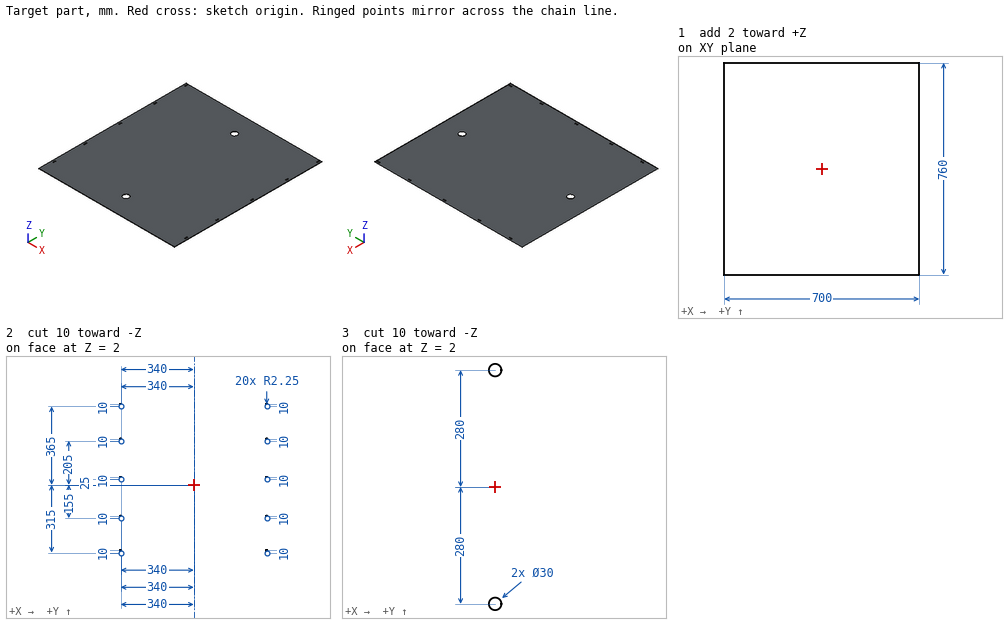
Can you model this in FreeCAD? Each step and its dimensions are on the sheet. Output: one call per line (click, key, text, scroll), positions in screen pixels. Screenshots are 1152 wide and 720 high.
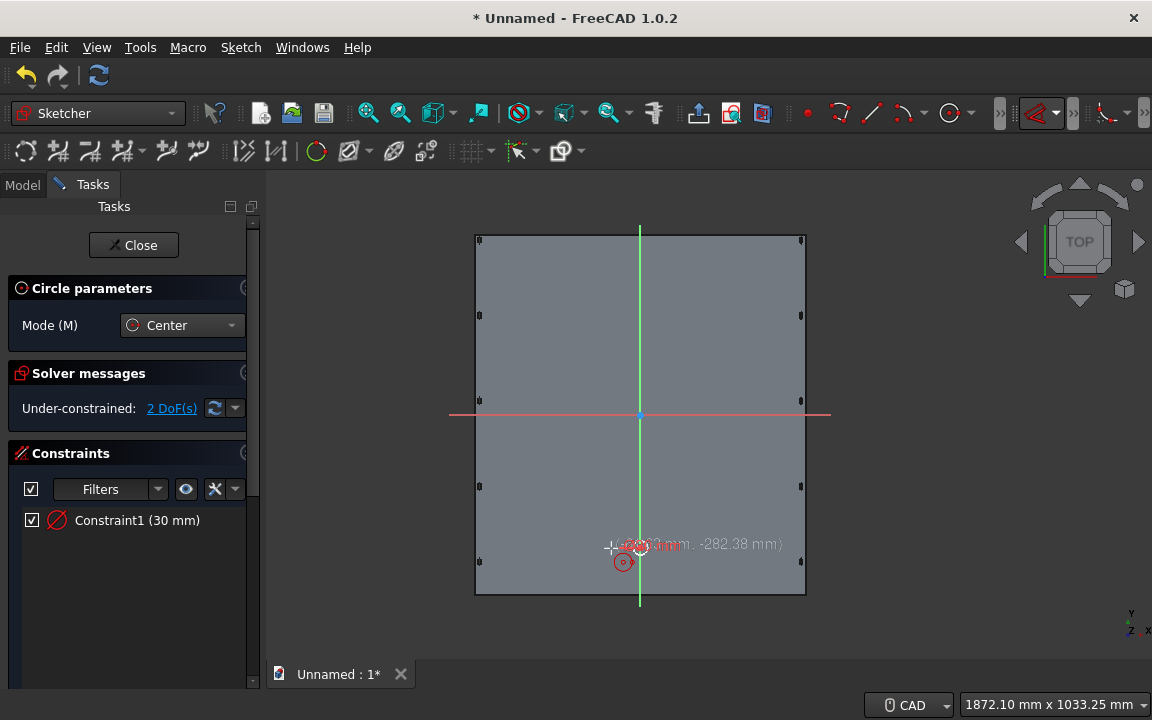
scroll(640, 283, up, 6)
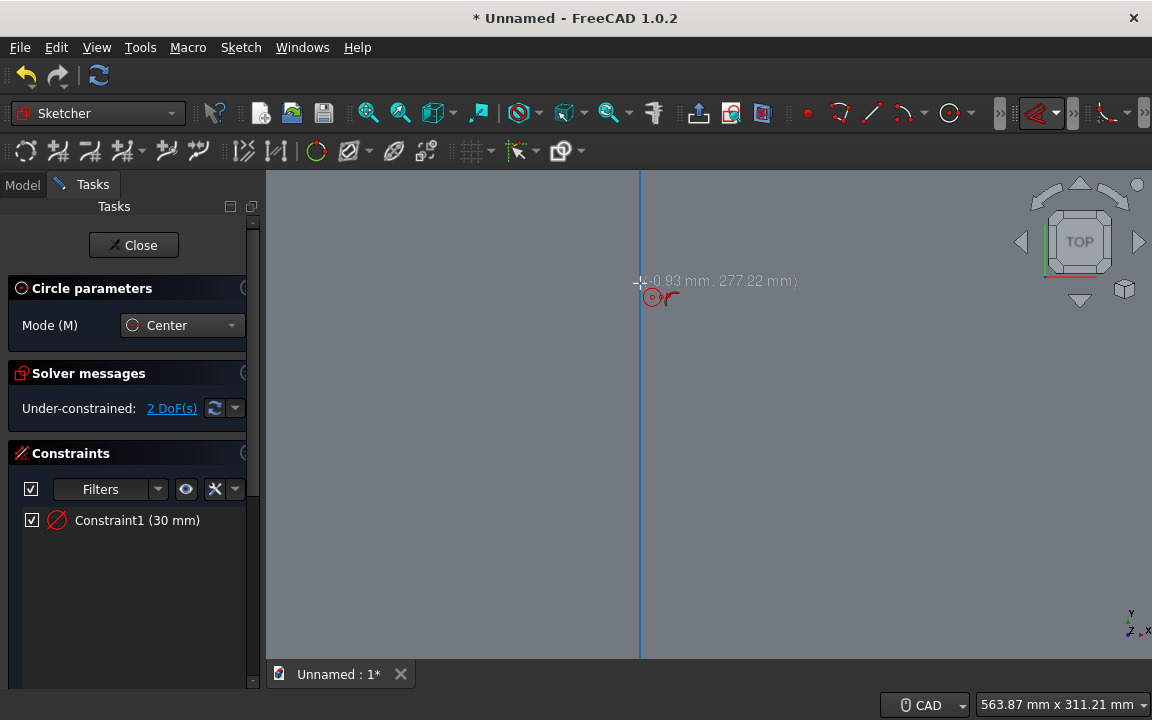
click(640, 281)
move(657, 265)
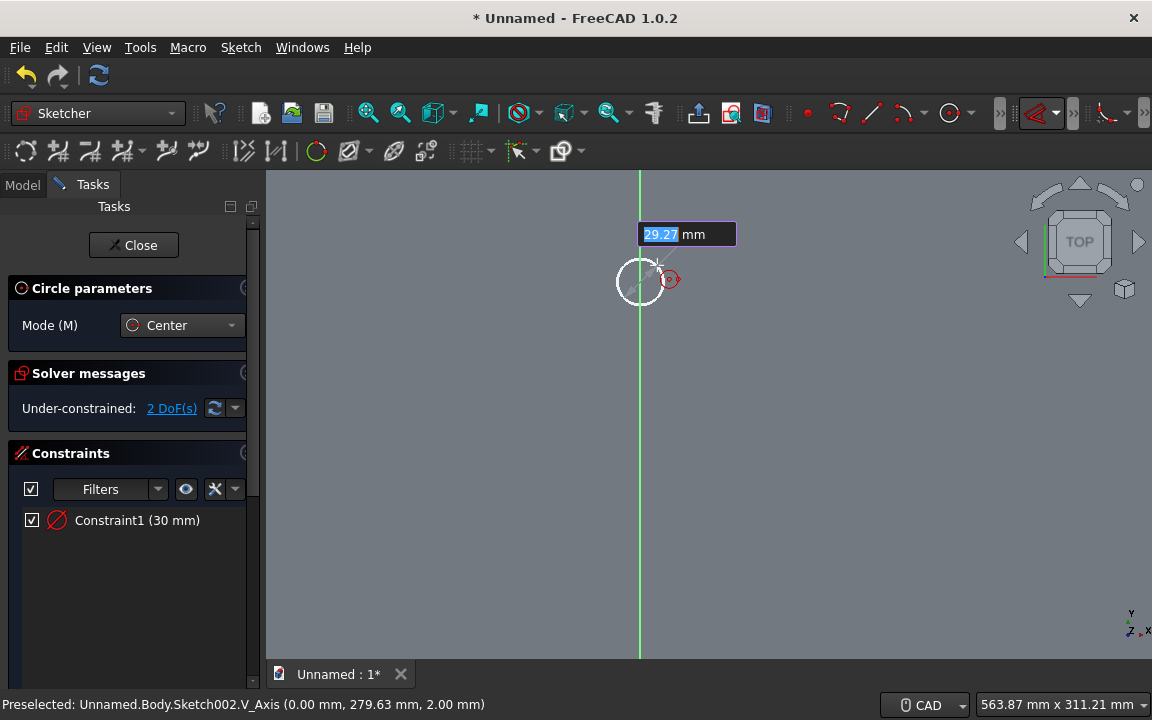
text(30)
key(Return)
key(Escape)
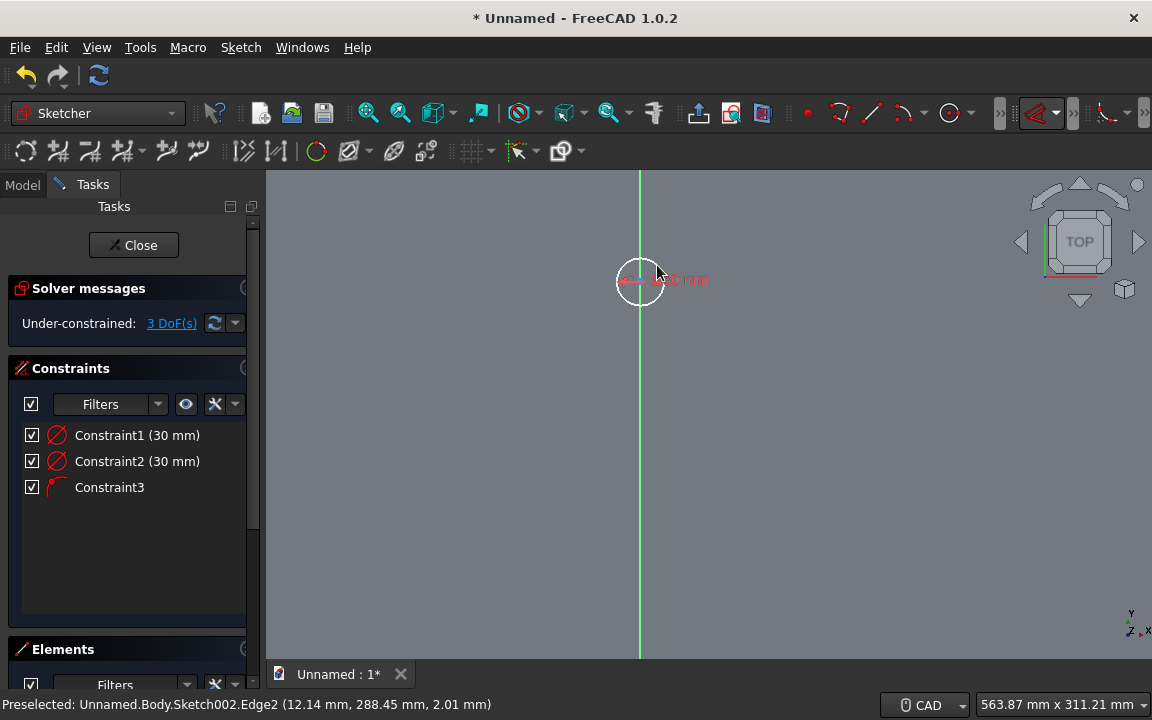
scroll(641, 282, down, 6)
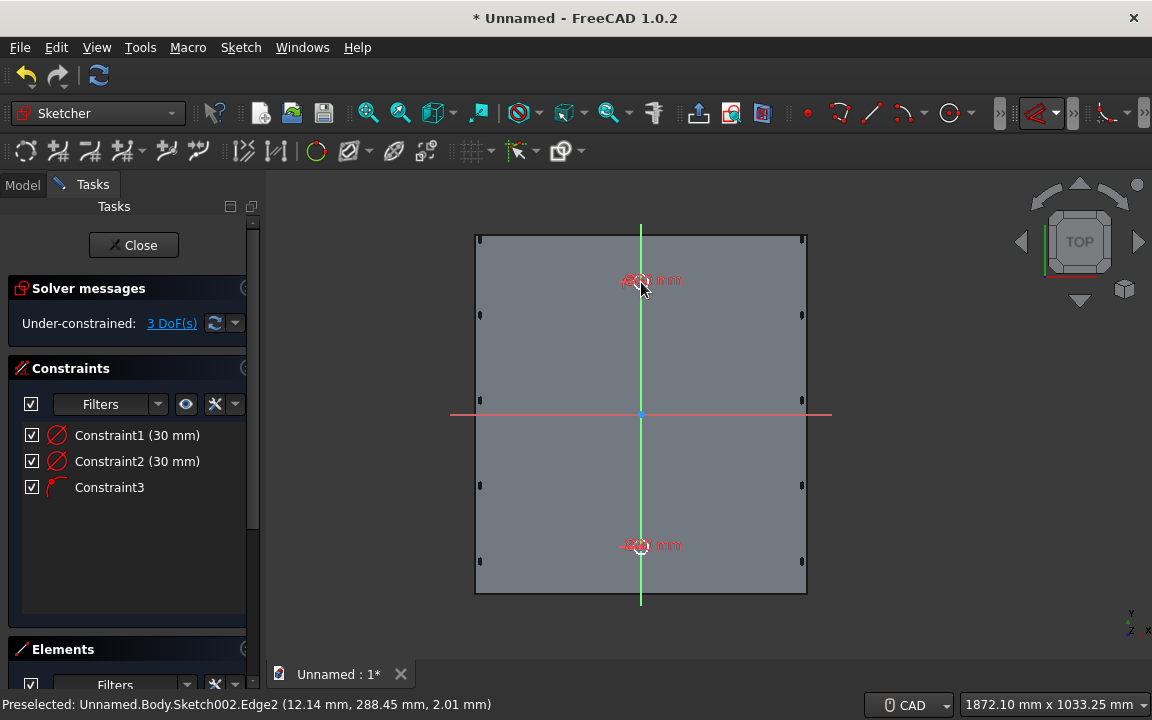
click(641, 547)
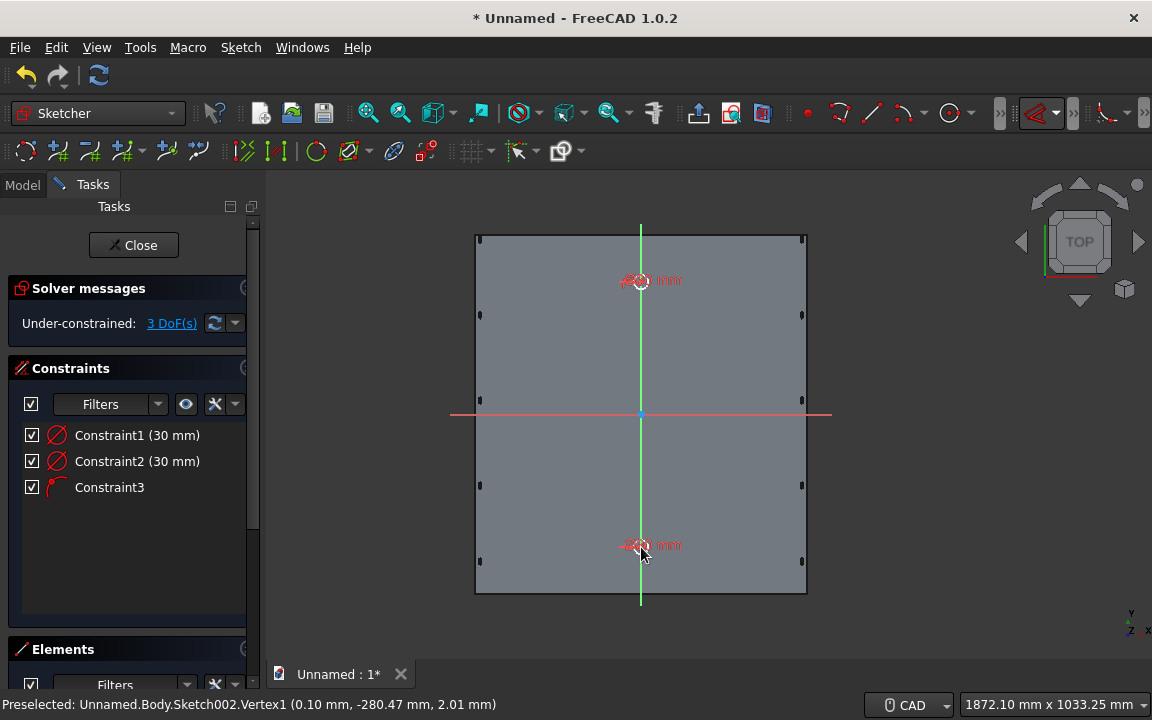
click(641, 600)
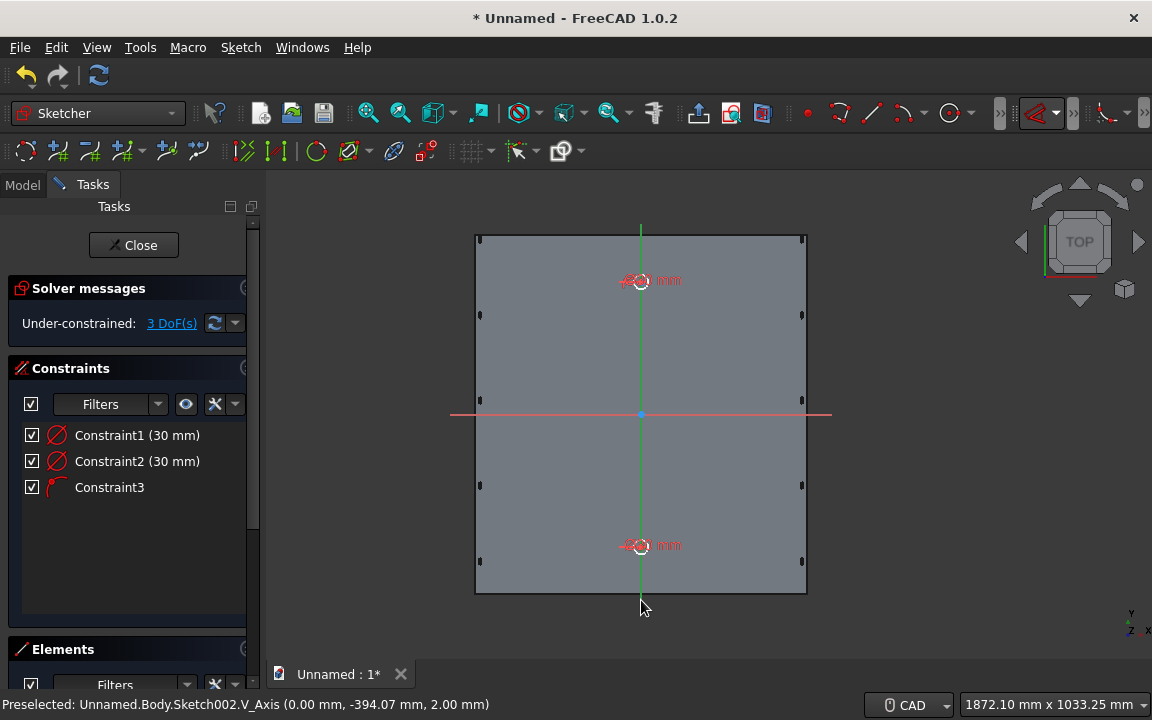
key(c)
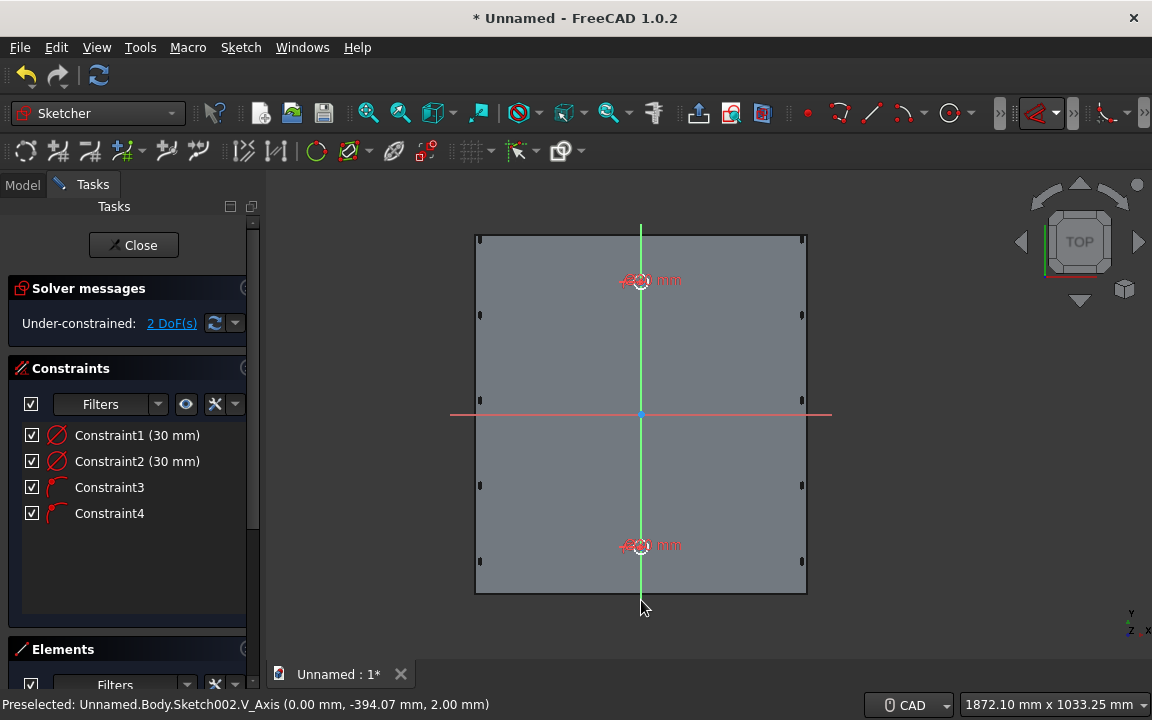
click(641, 547)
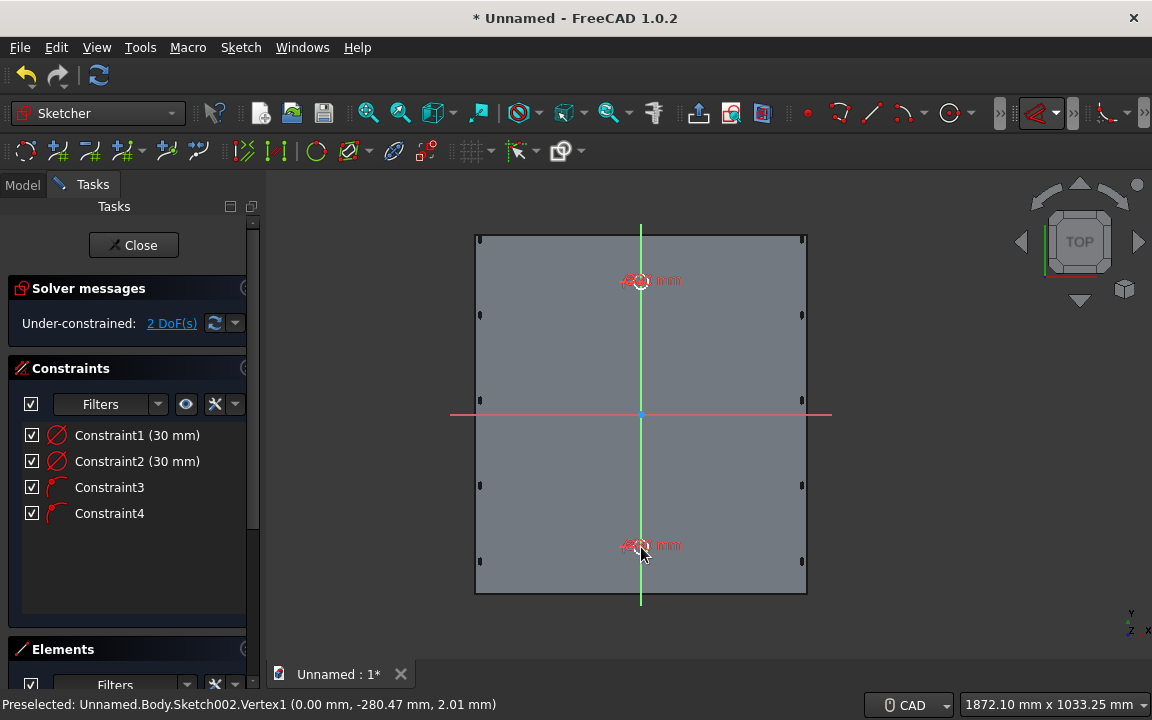
click(1058, 114)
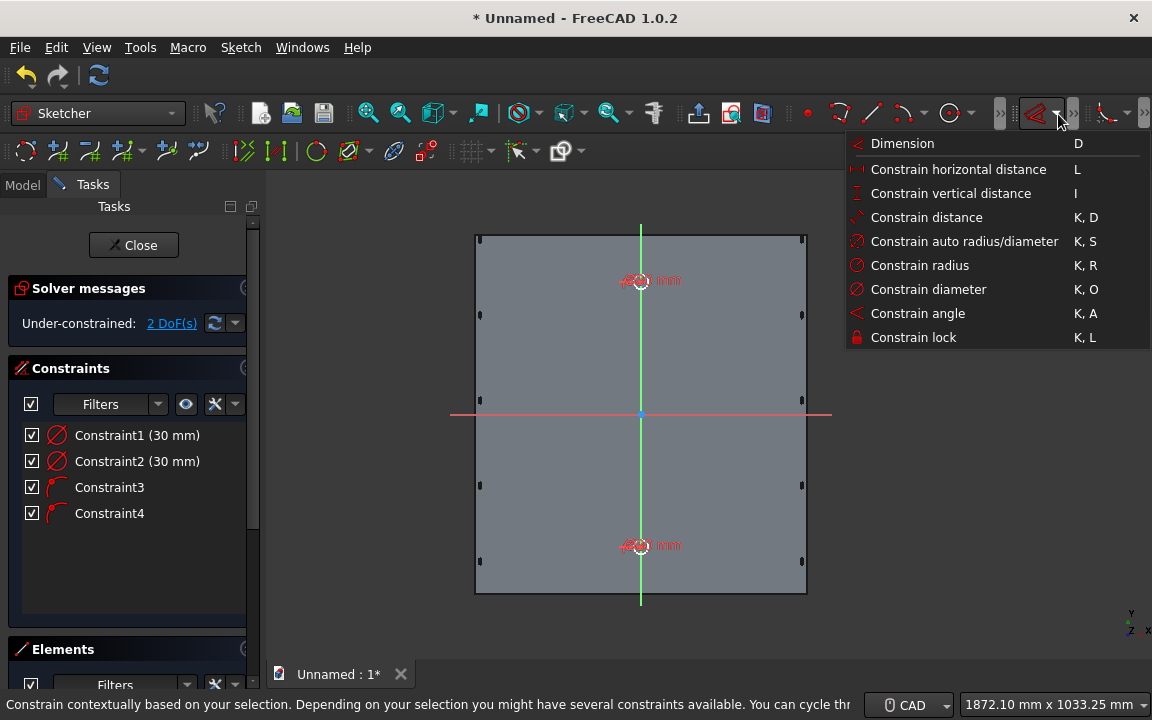
click(998, 193)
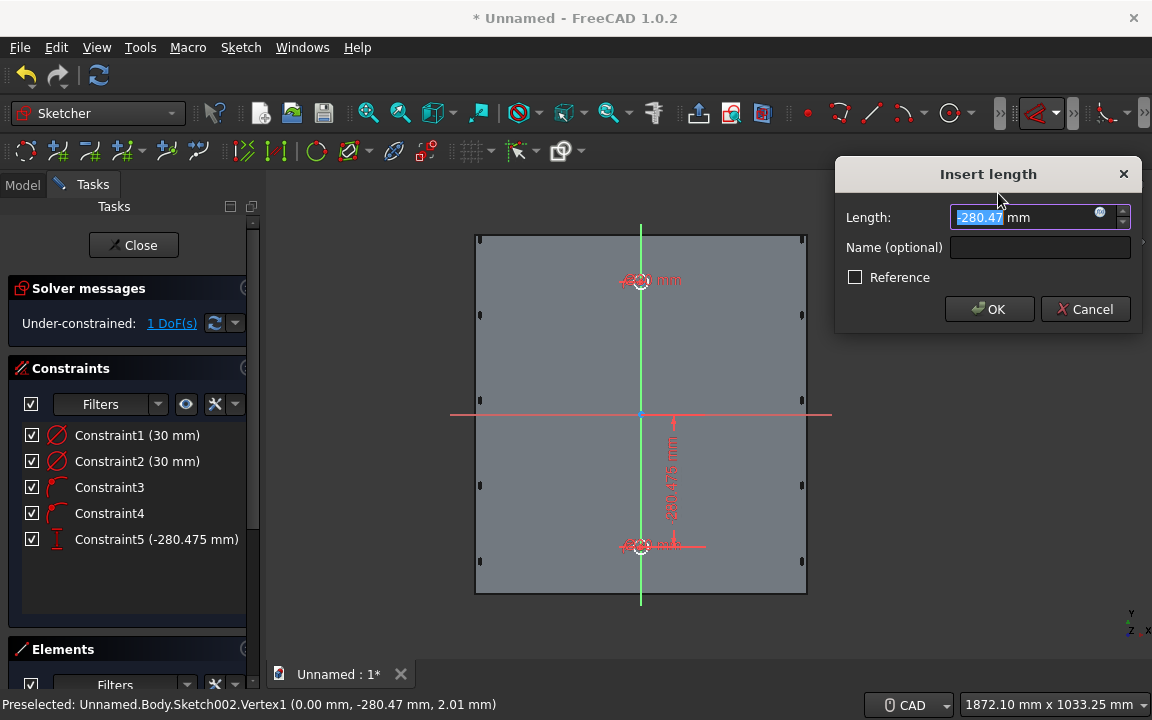
text(-280)
key(Return)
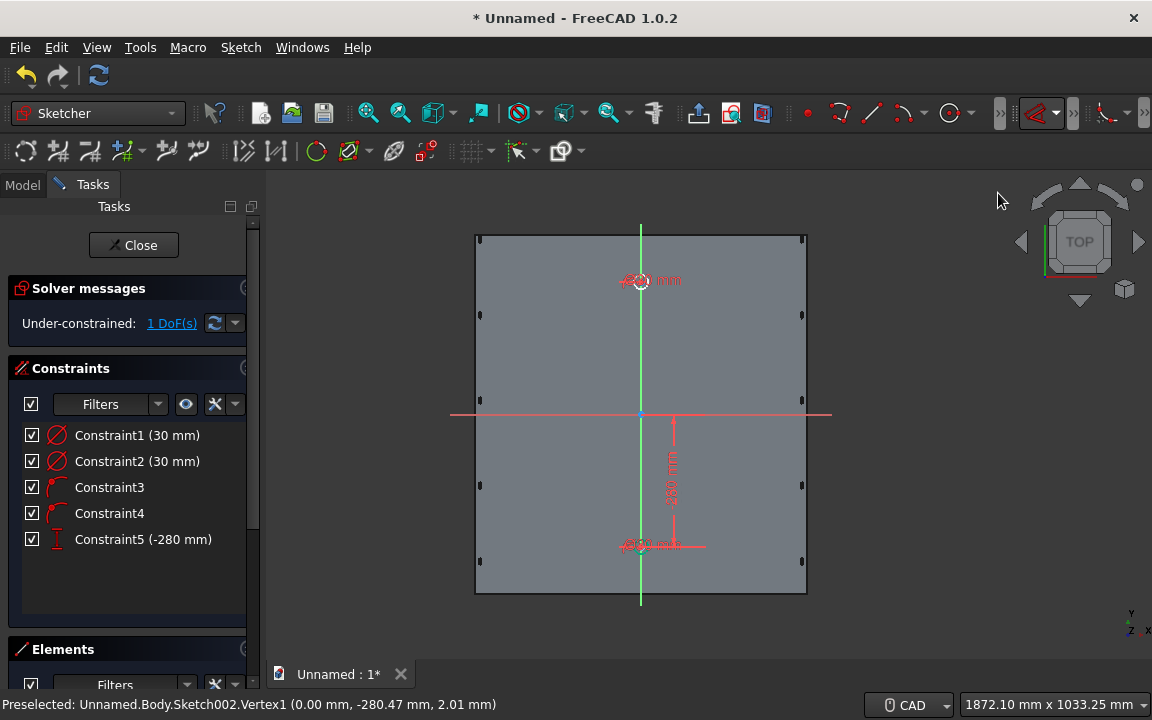
click(641, 282)